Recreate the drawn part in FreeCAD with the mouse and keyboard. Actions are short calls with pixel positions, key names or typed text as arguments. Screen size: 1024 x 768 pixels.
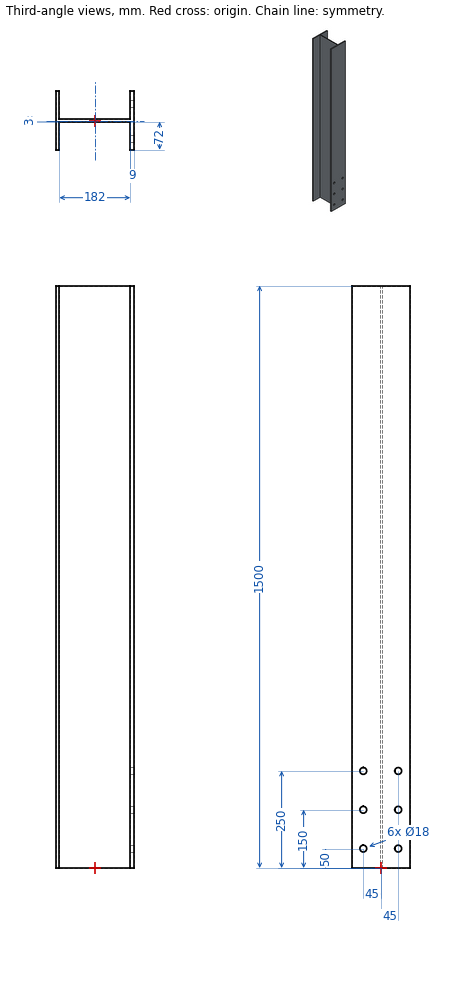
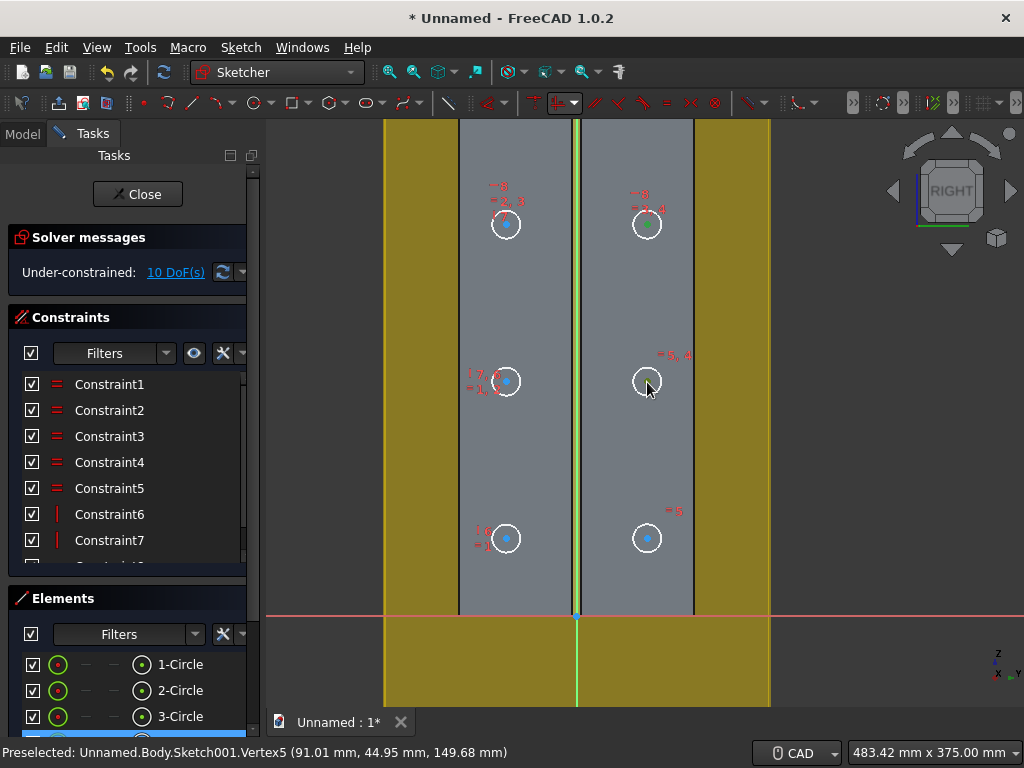
click(576, 104)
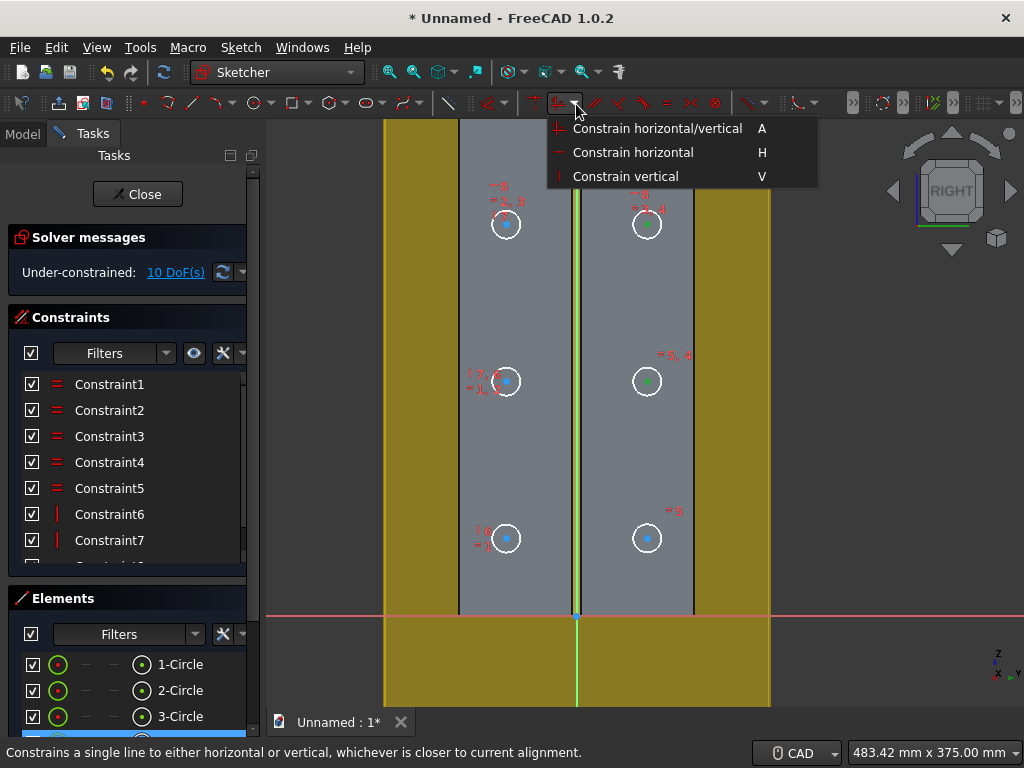
click(683, 176)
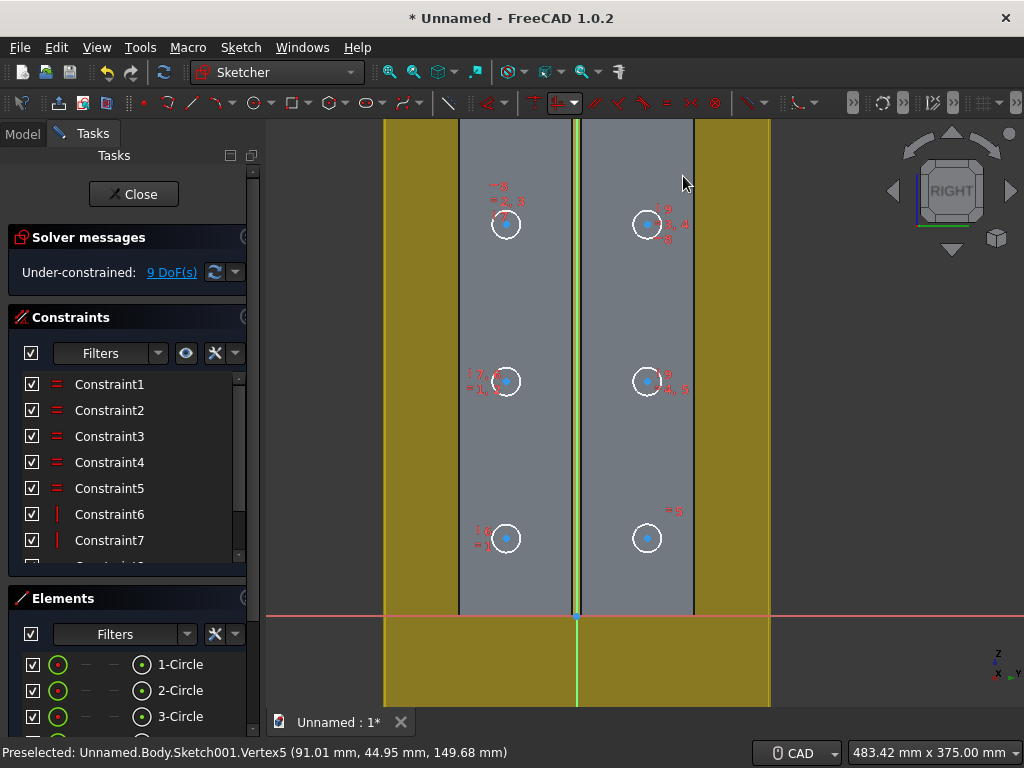
click(506, 382)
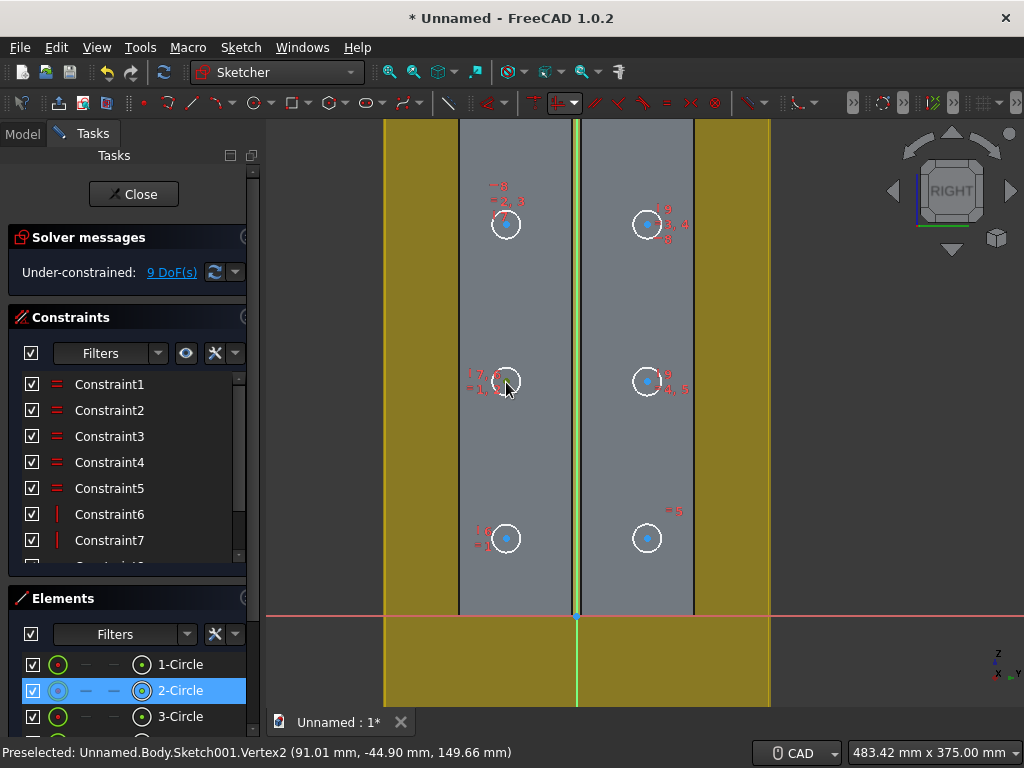
click(647, 382)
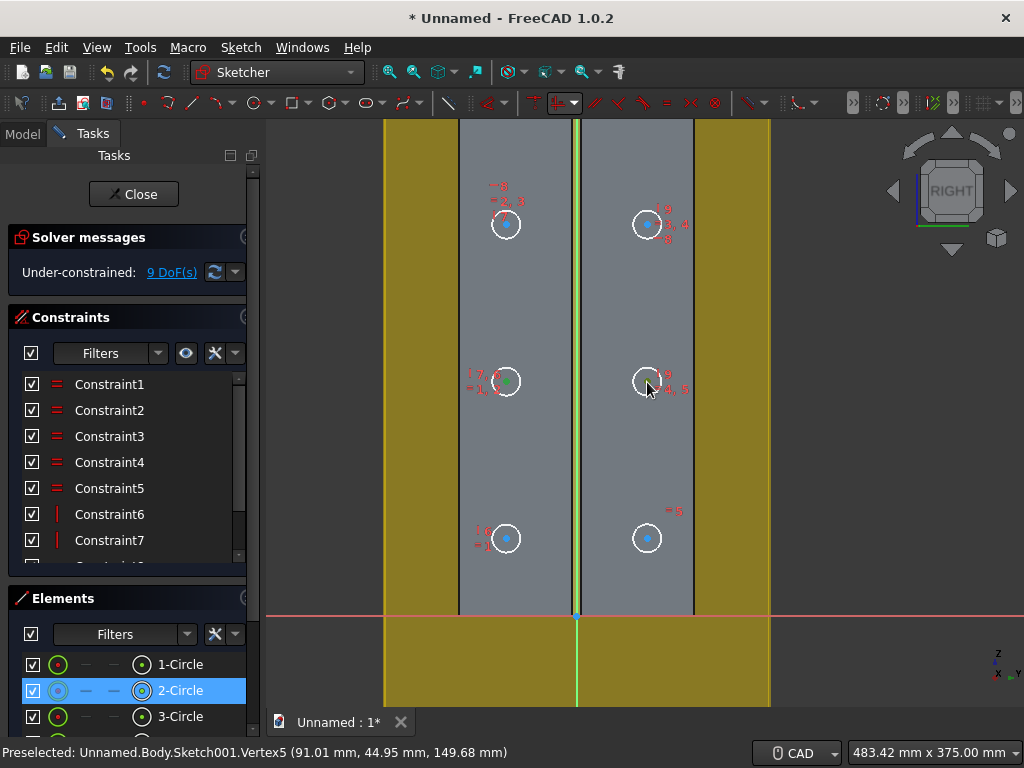
click(576, 104)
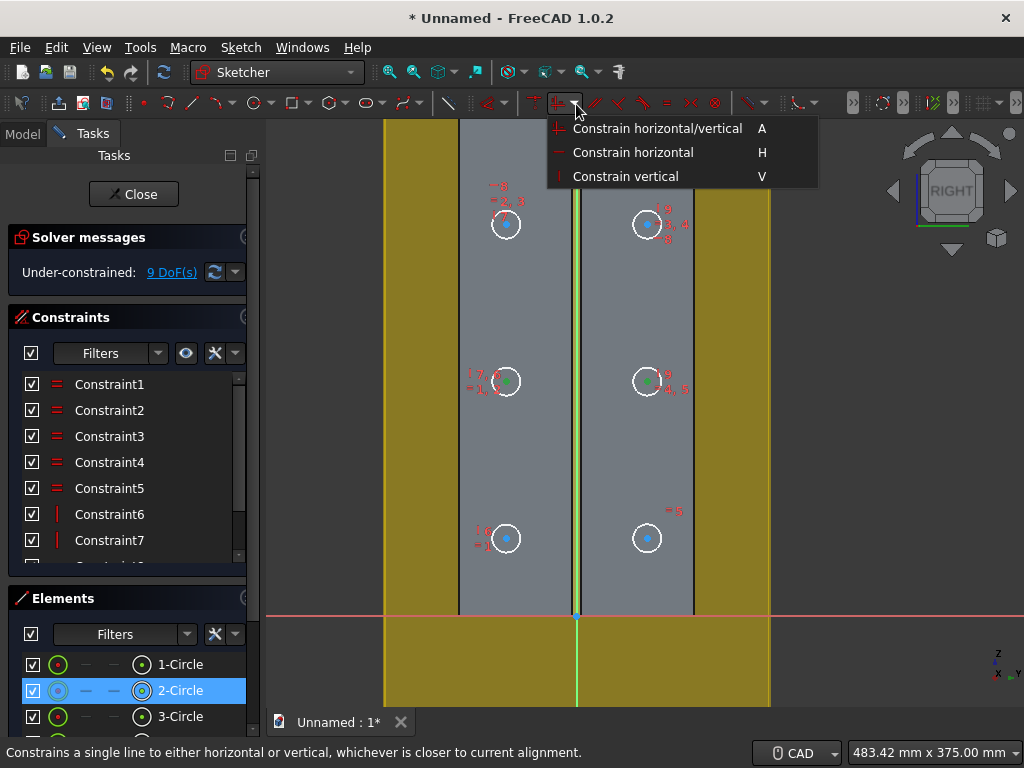
click(683, 152)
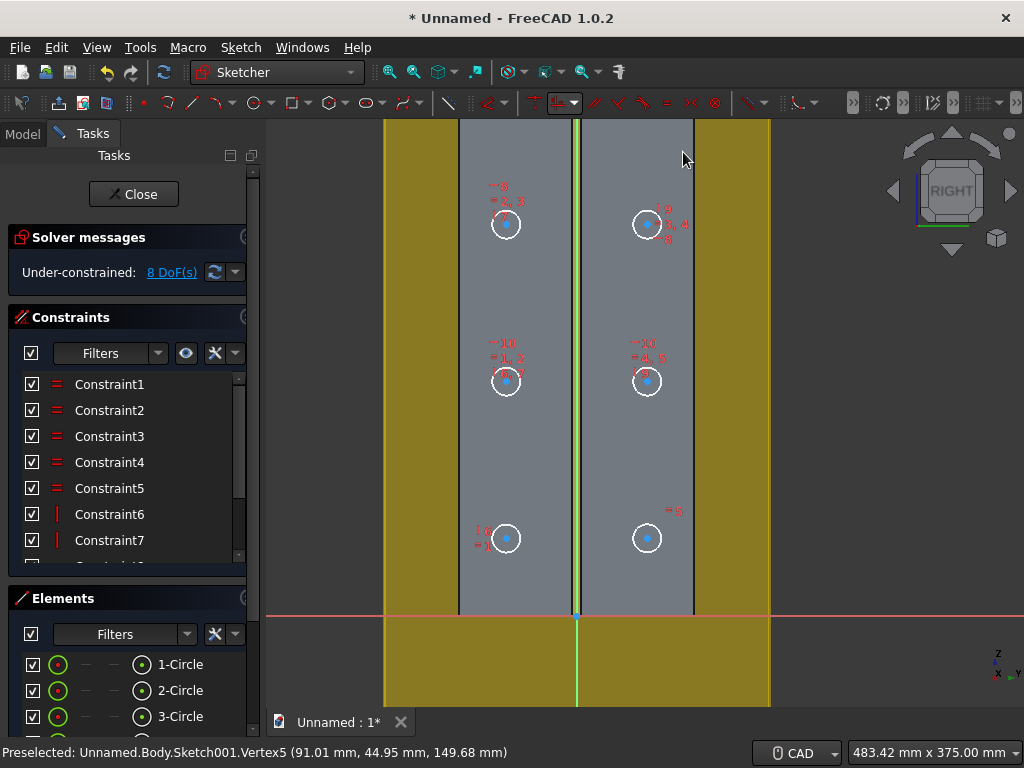
click(647, 382)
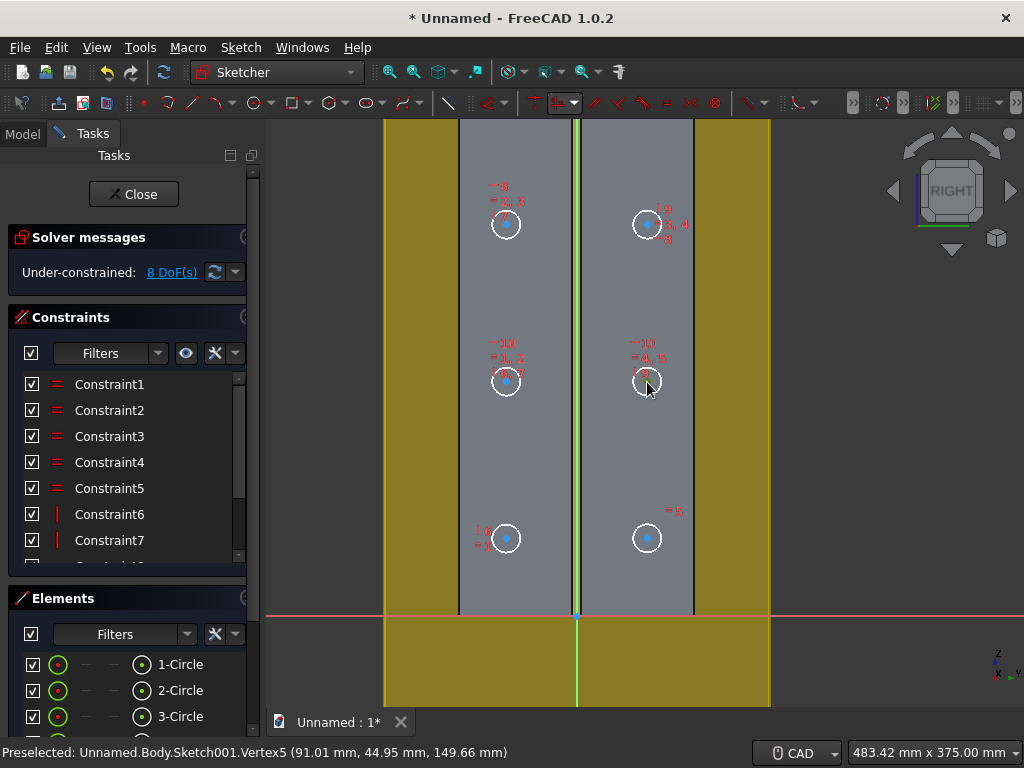
click(647, 538)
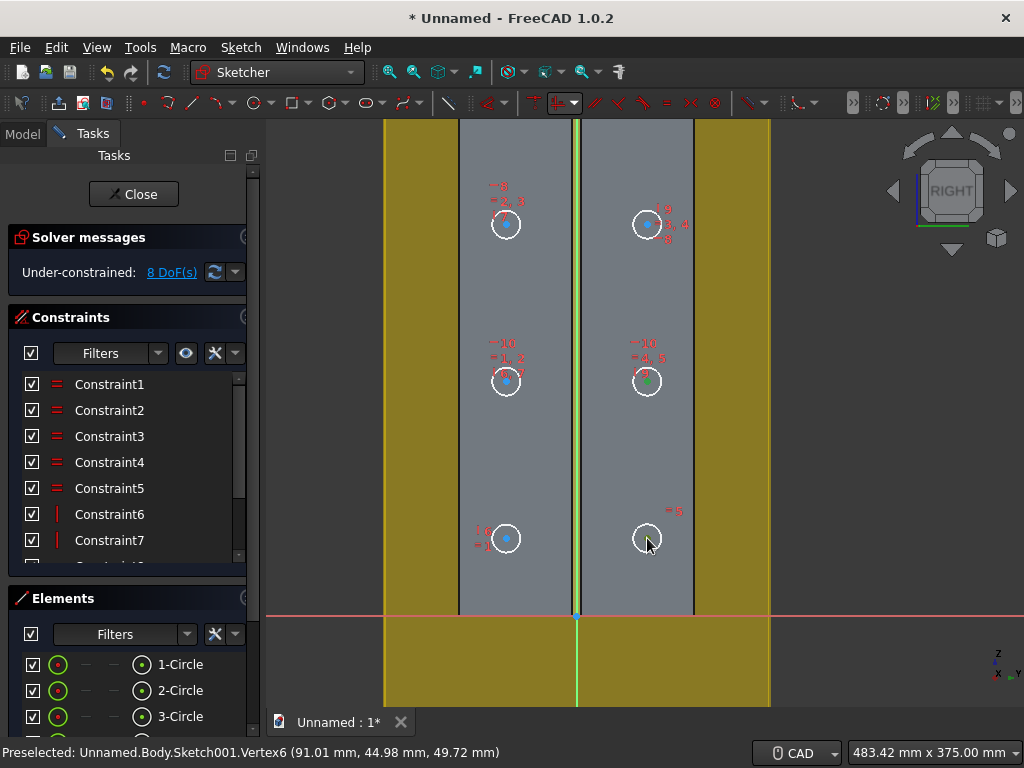
click(576, 104)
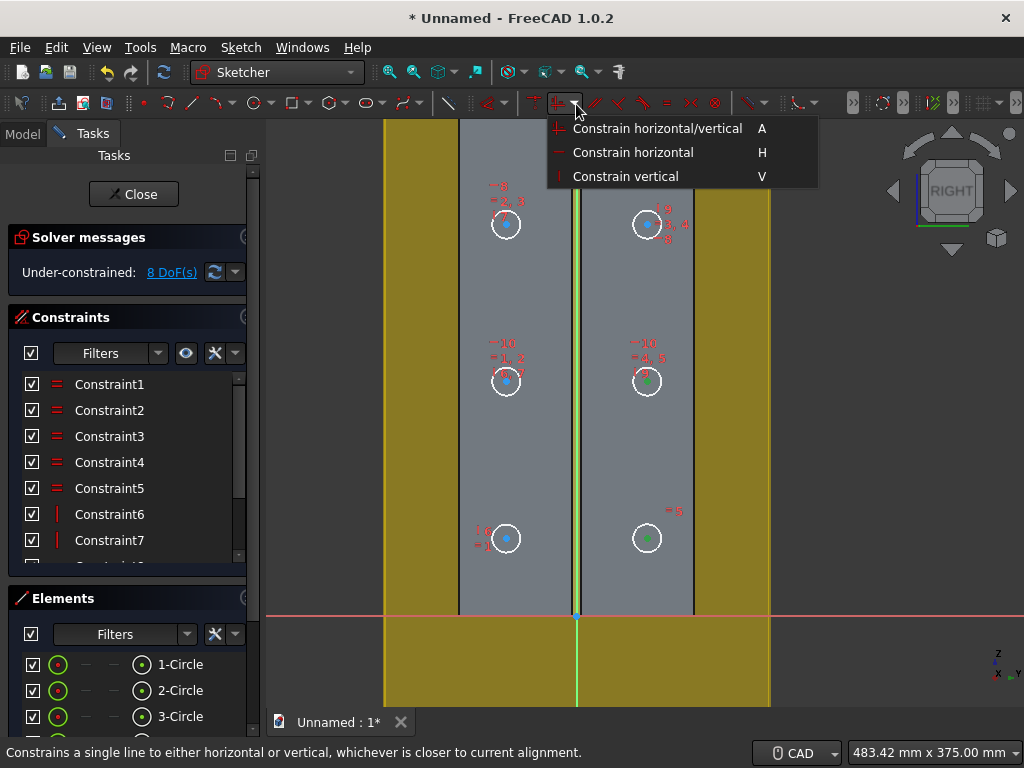
click(683, 176)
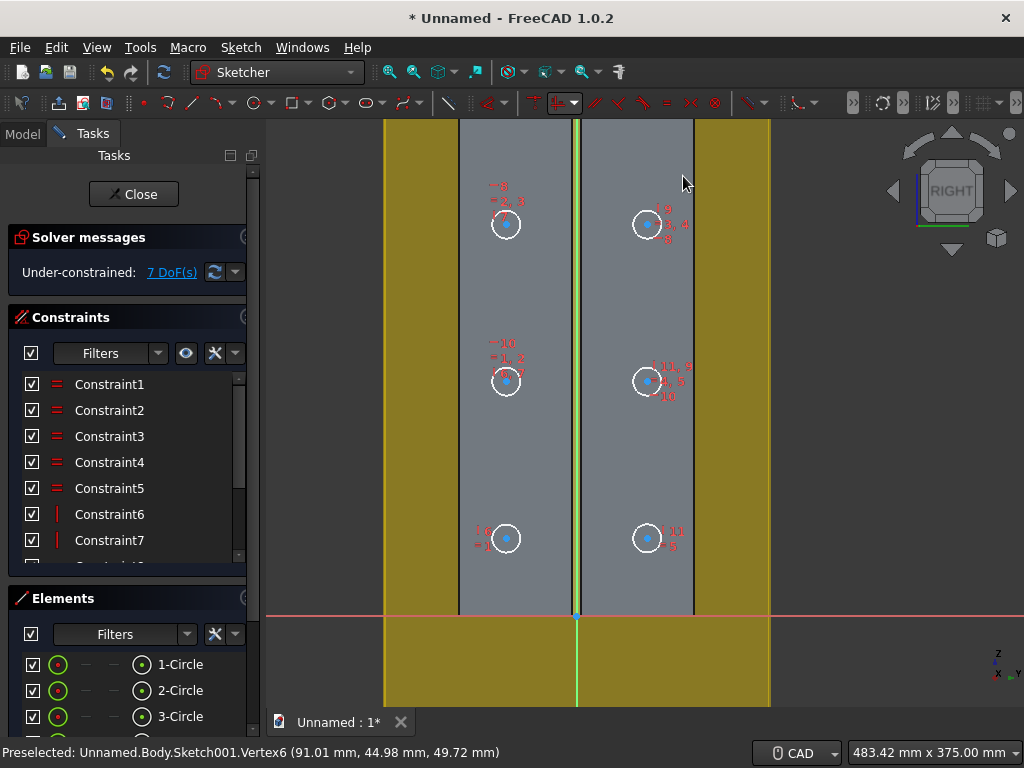
click(506, 539)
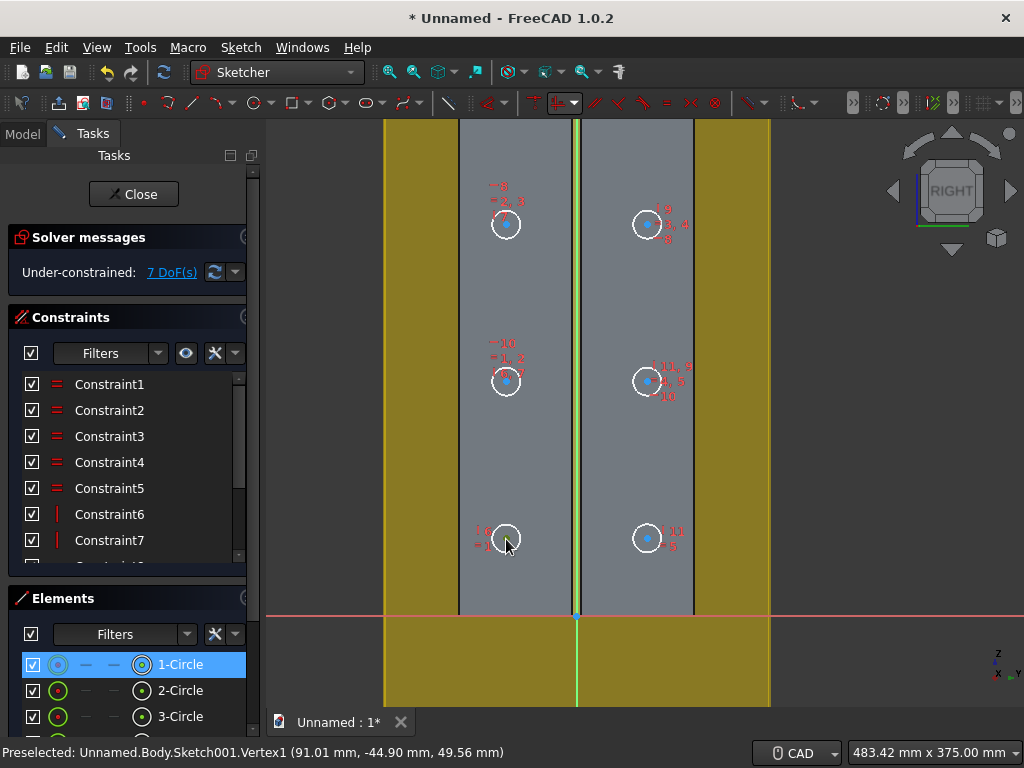
click(647, 538)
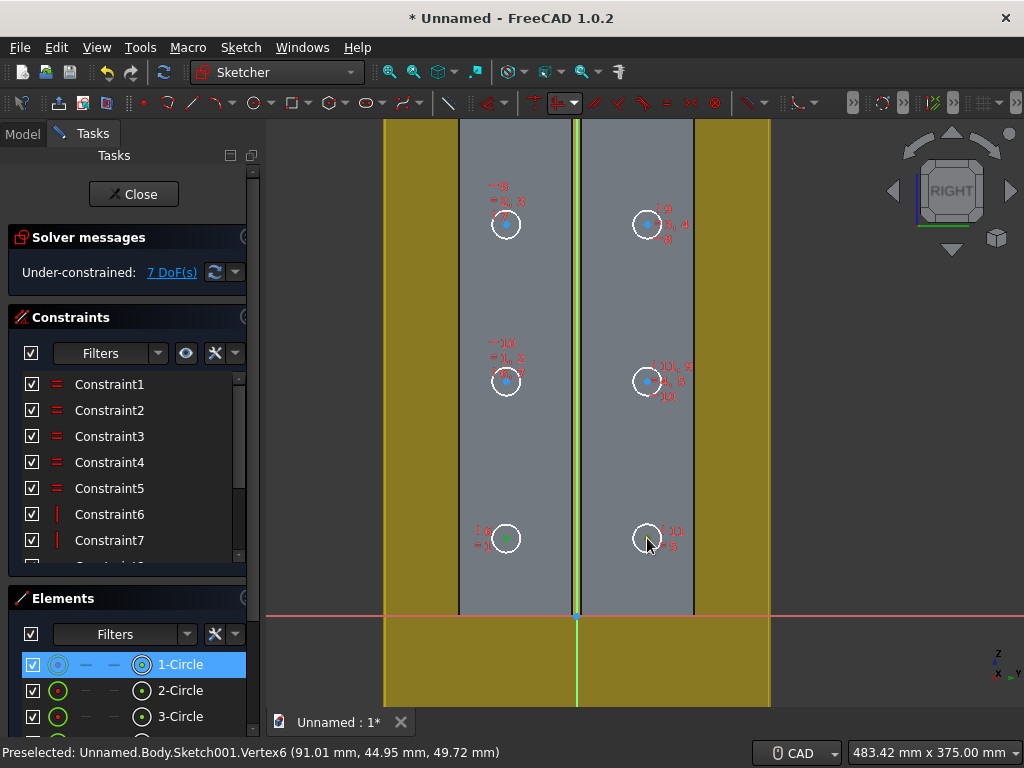
key(h)